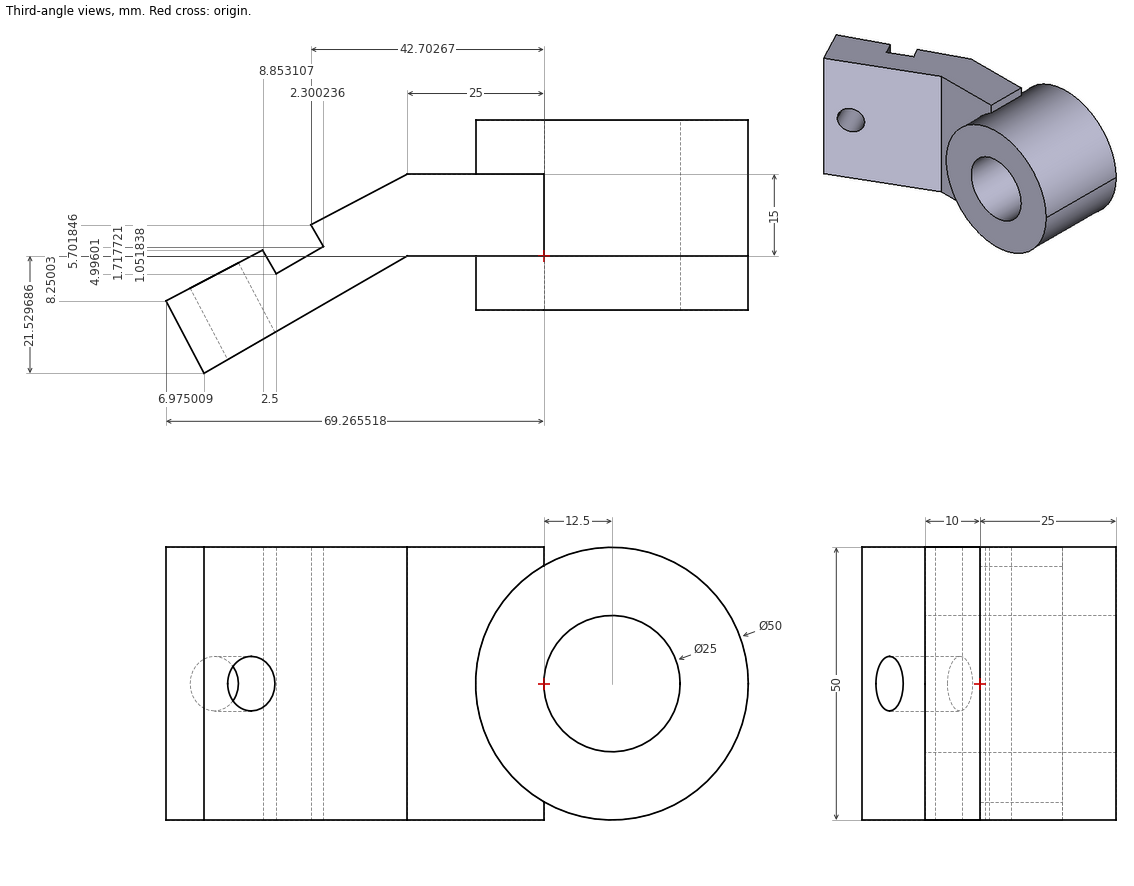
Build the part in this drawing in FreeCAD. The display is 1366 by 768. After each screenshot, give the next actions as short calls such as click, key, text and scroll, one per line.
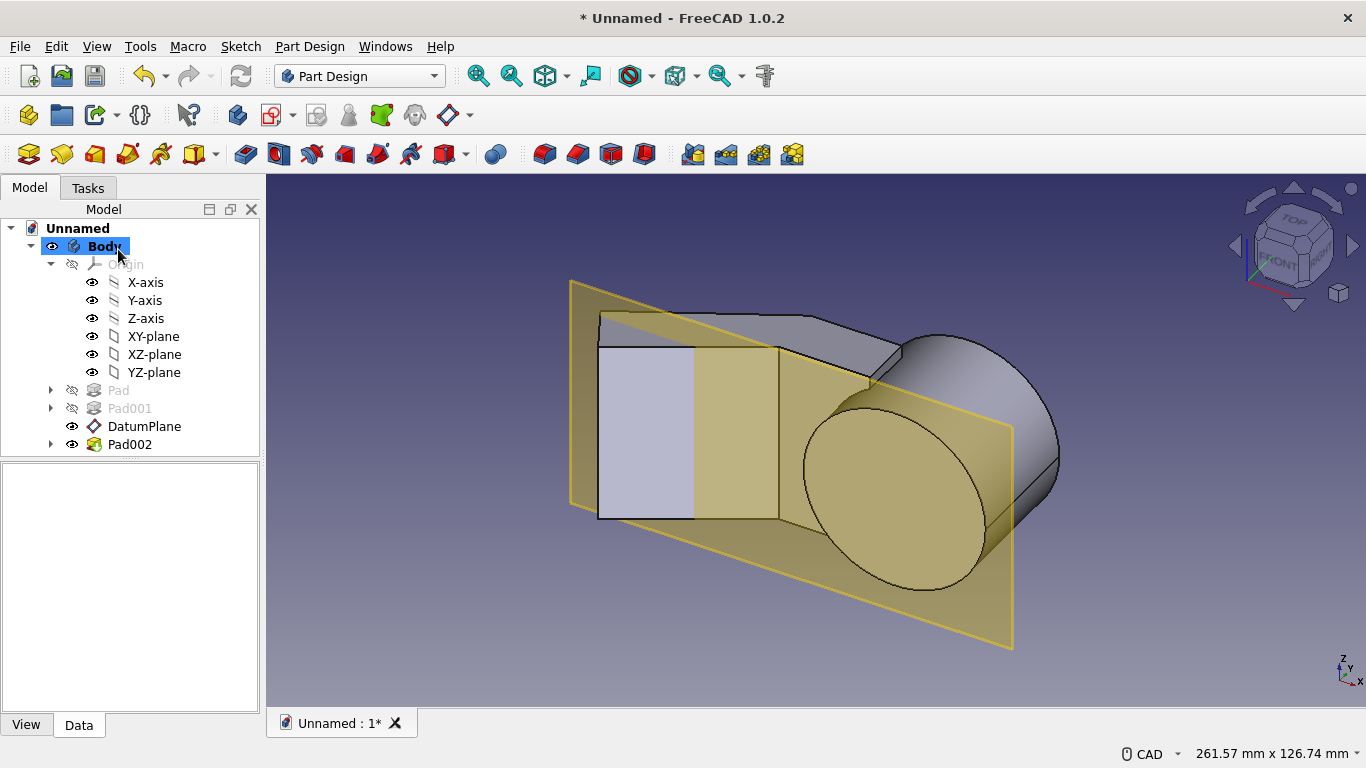
click(117, 426)
key(space)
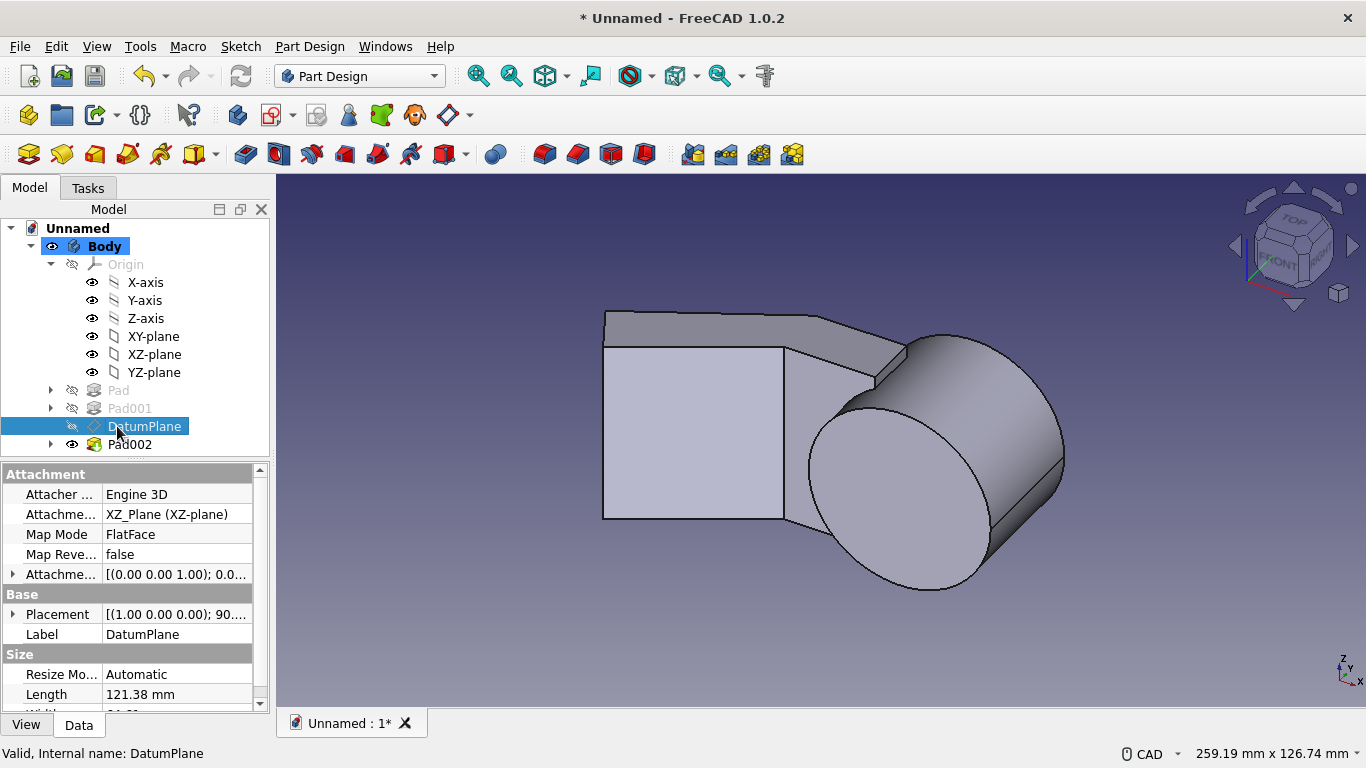
click(900, 498)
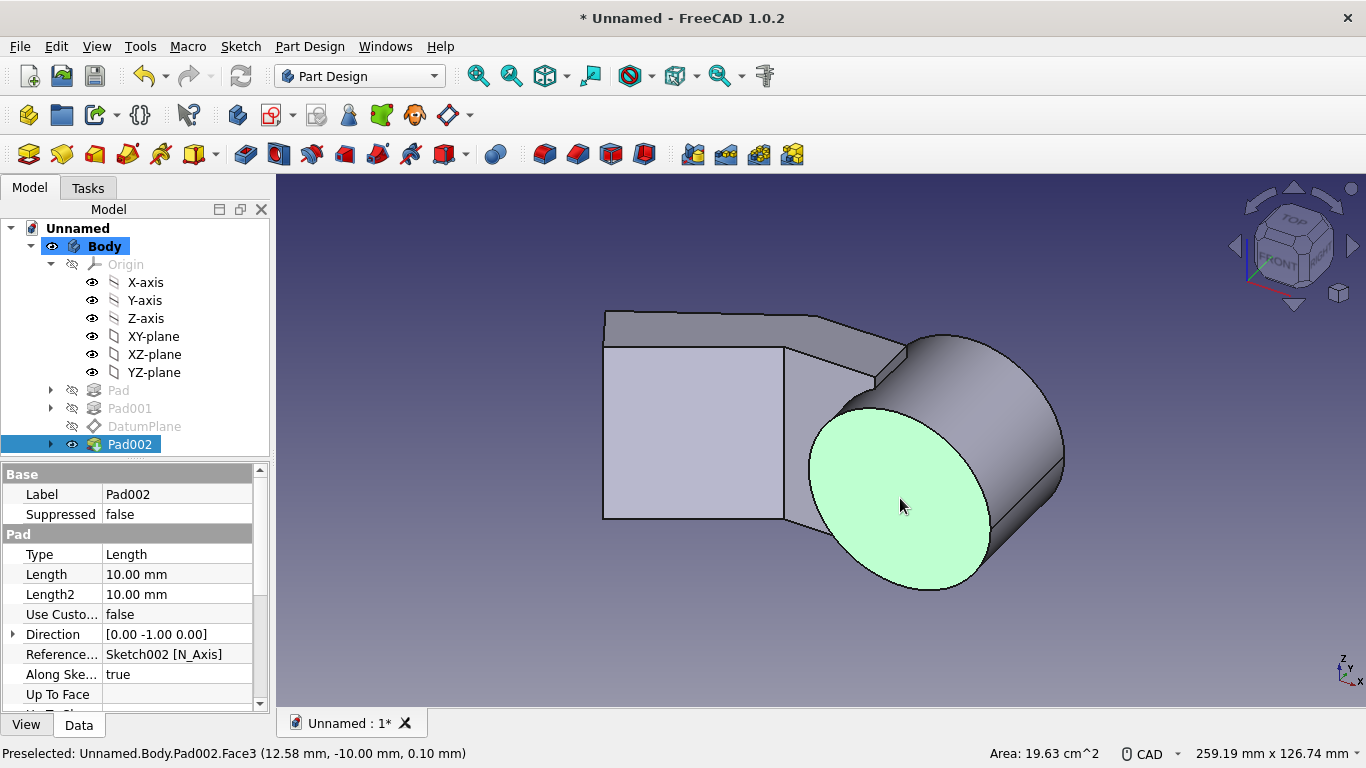
click(270, 116)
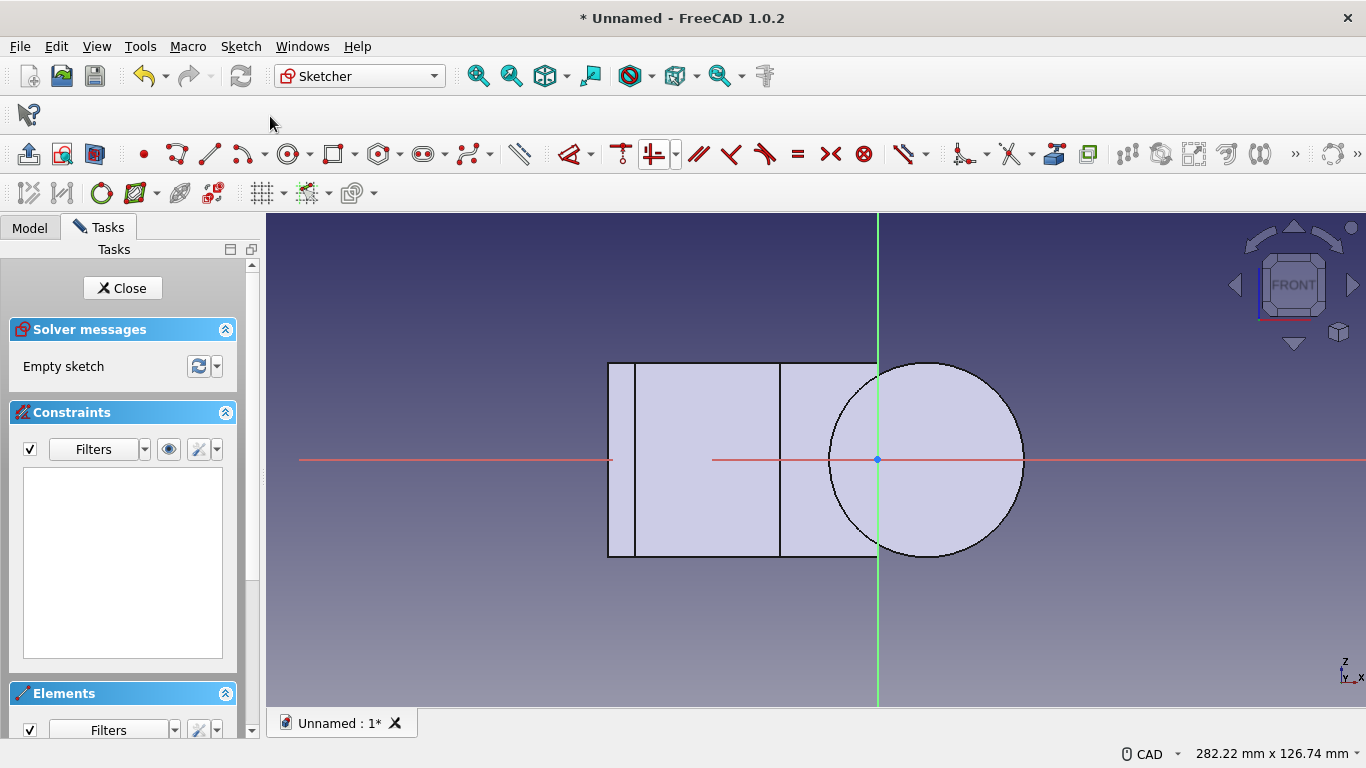
scroll(1004, 460, up, 6)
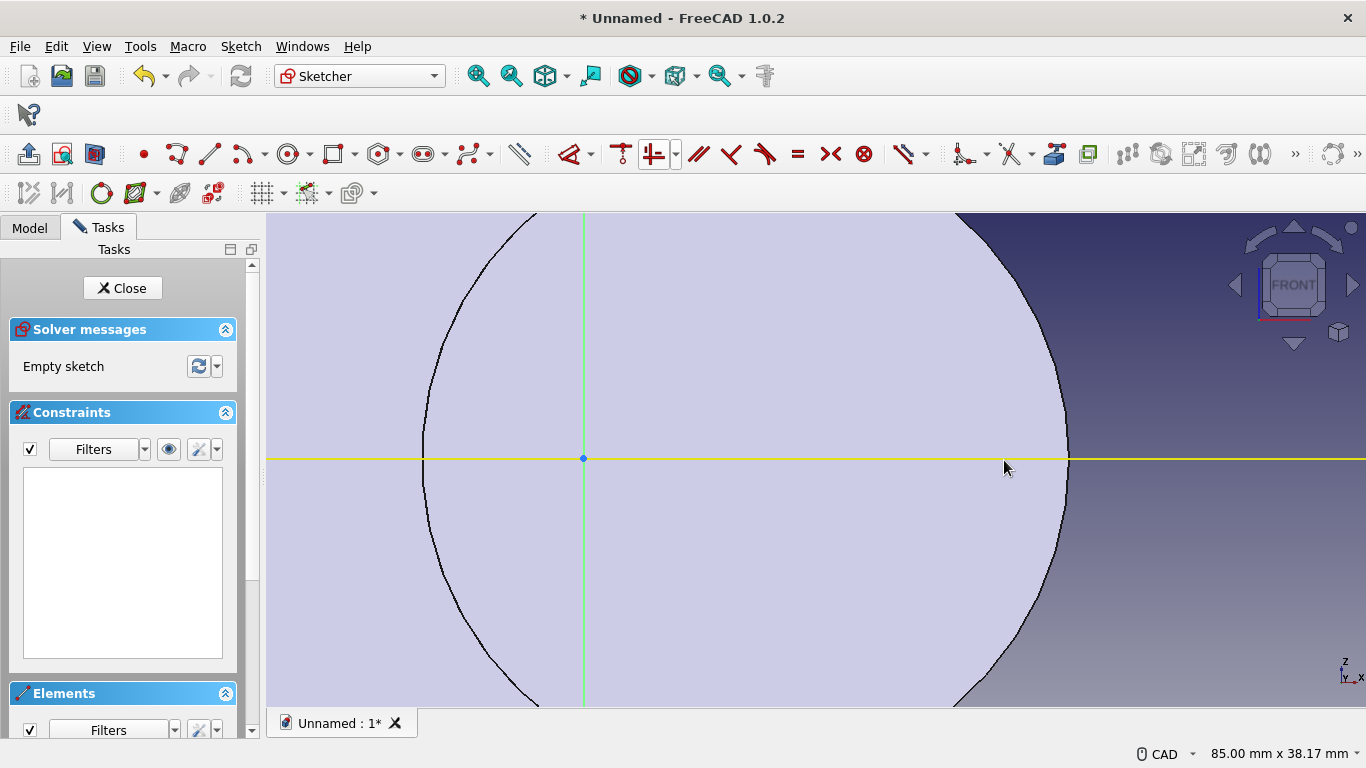
click(288, 154)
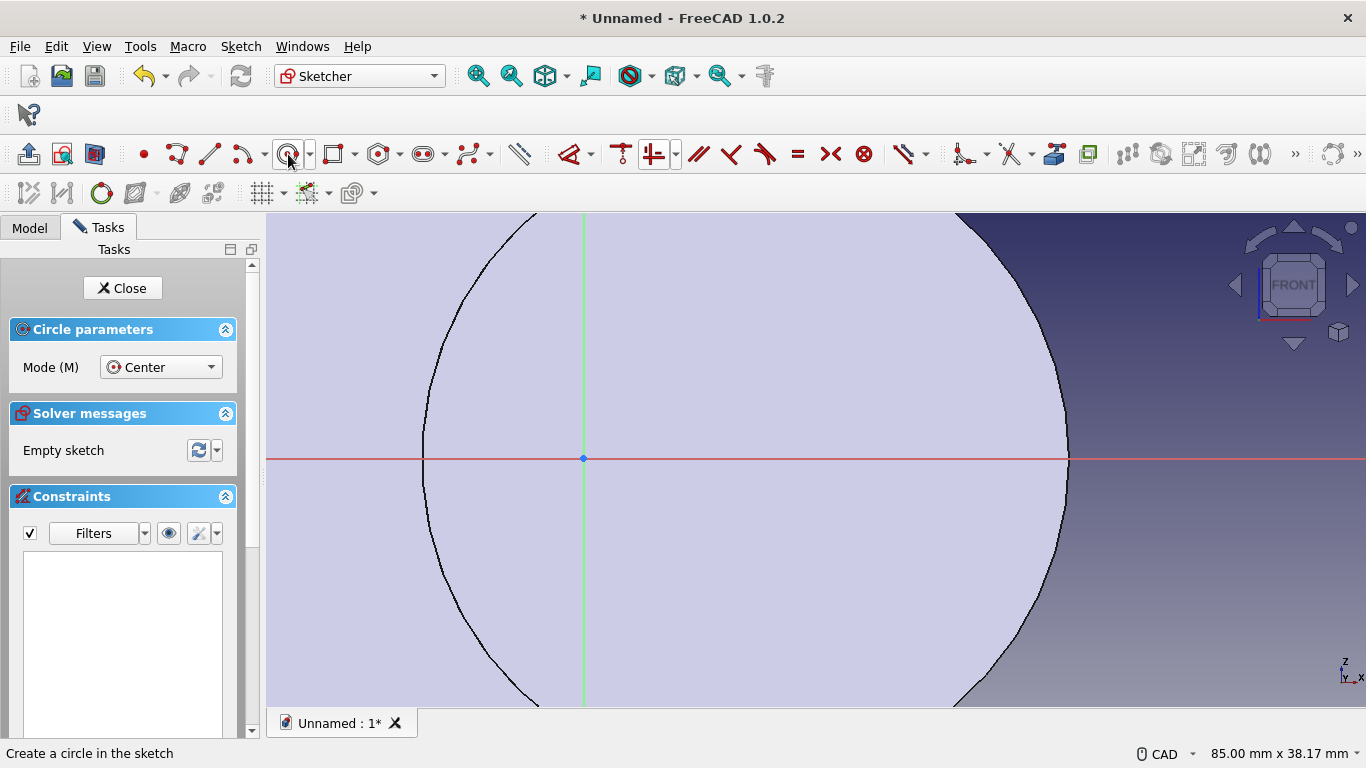
click(746, 459)
click(860, 344)
key(Escape)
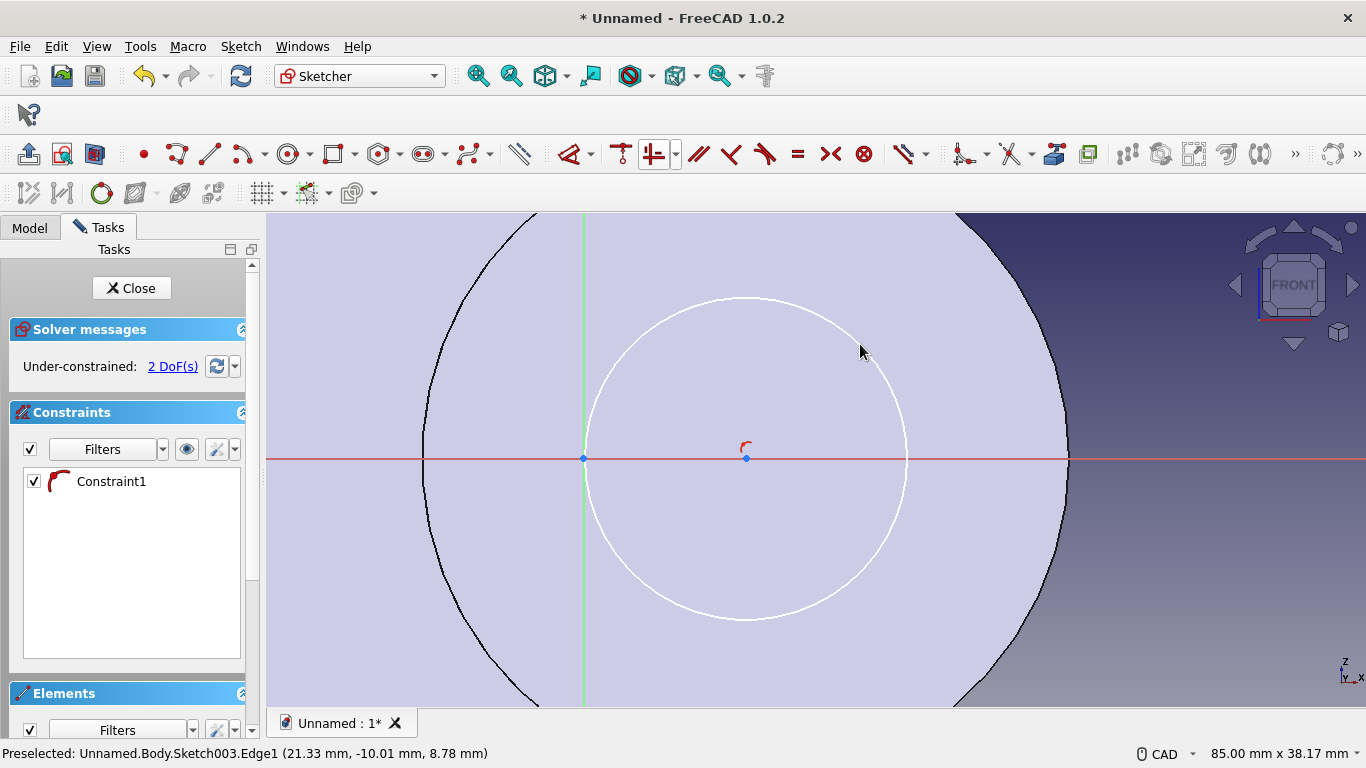
click(568, 154)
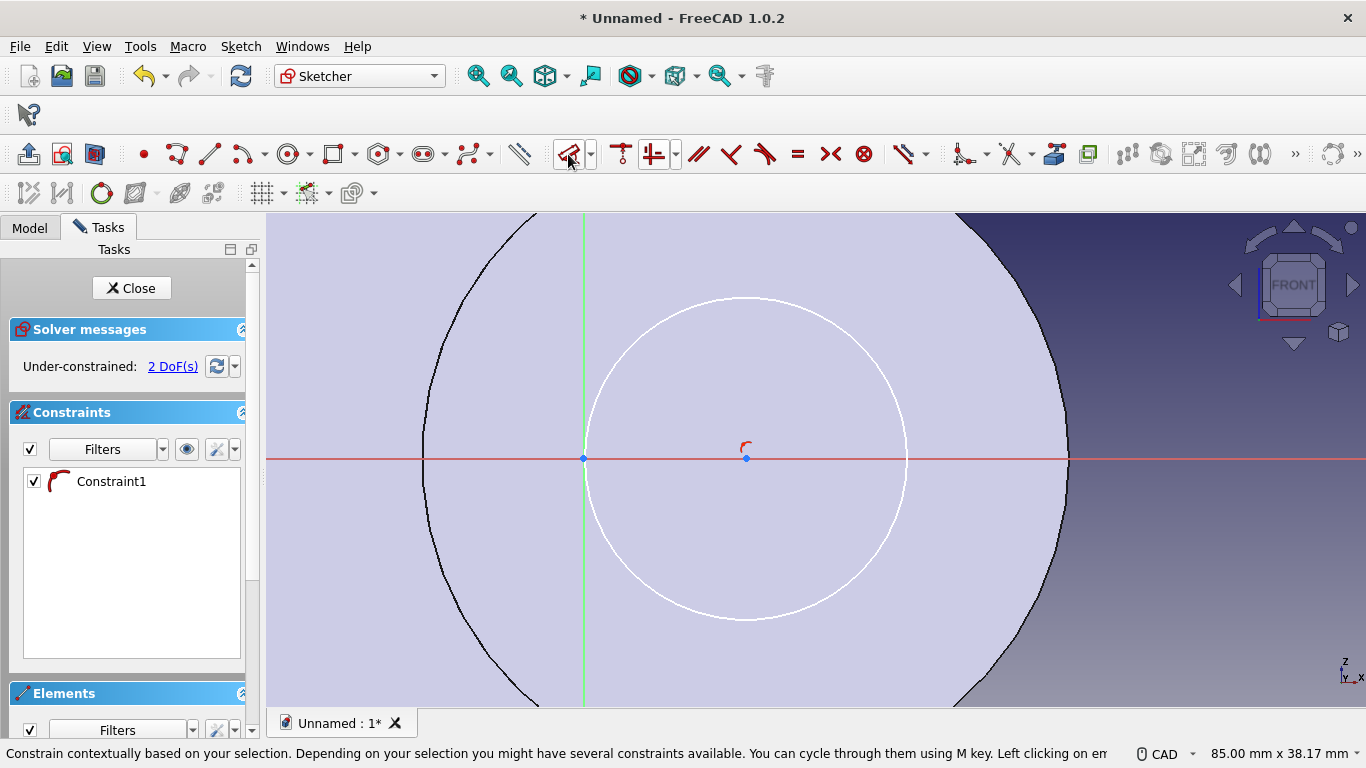
click(860, 345)
click(883, 322)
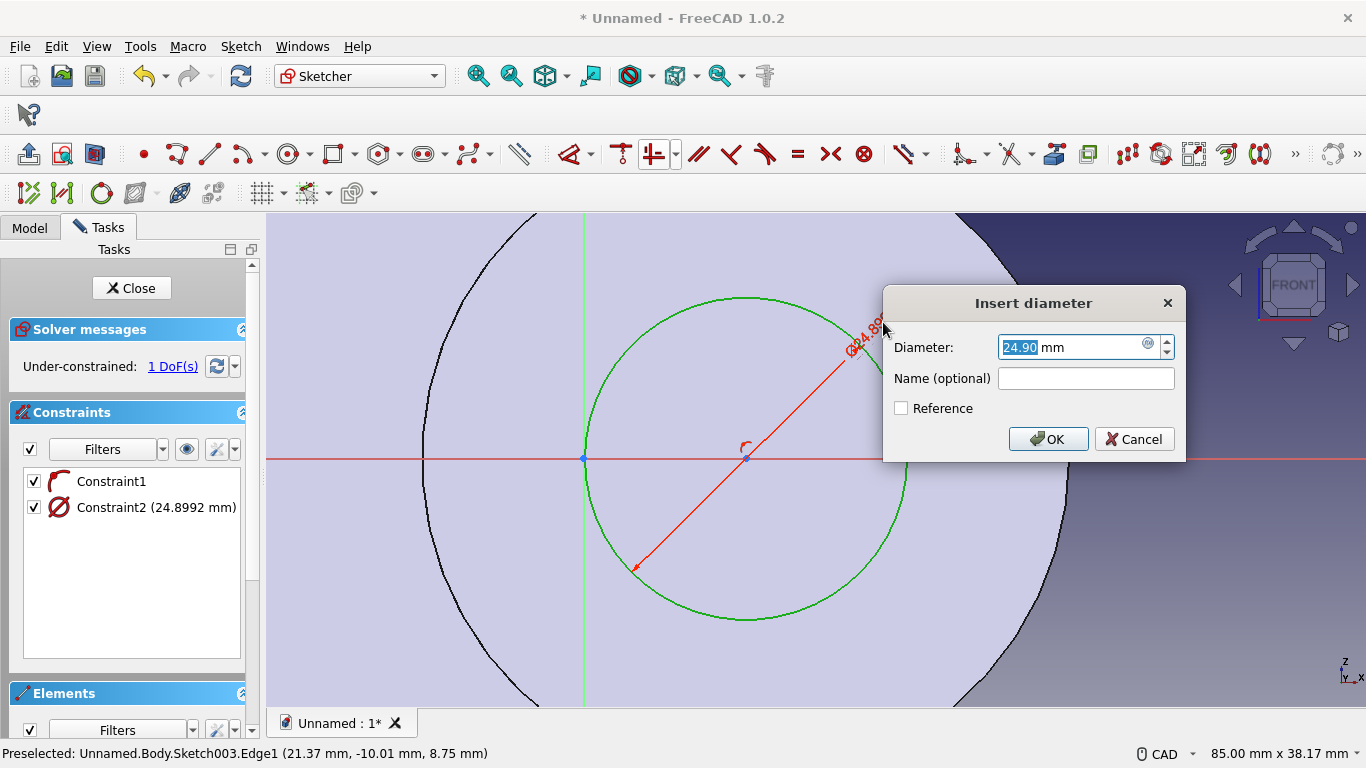
text(25)
key(Return)